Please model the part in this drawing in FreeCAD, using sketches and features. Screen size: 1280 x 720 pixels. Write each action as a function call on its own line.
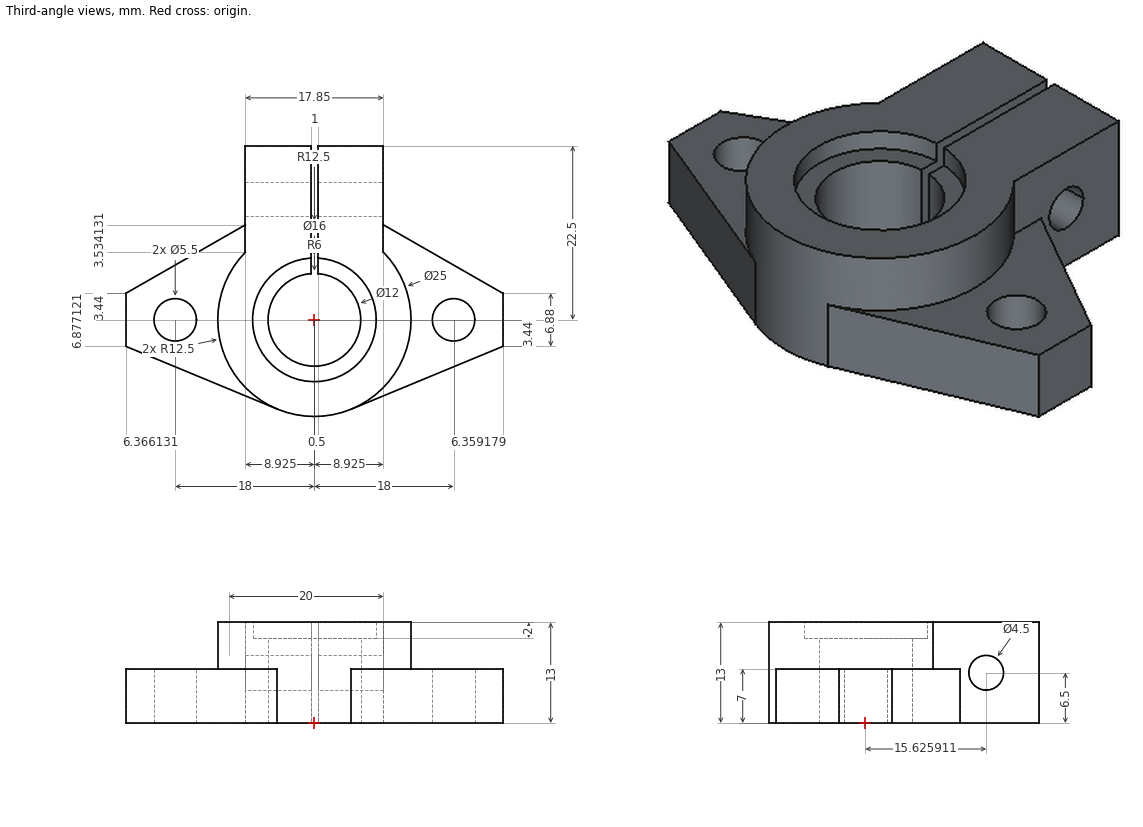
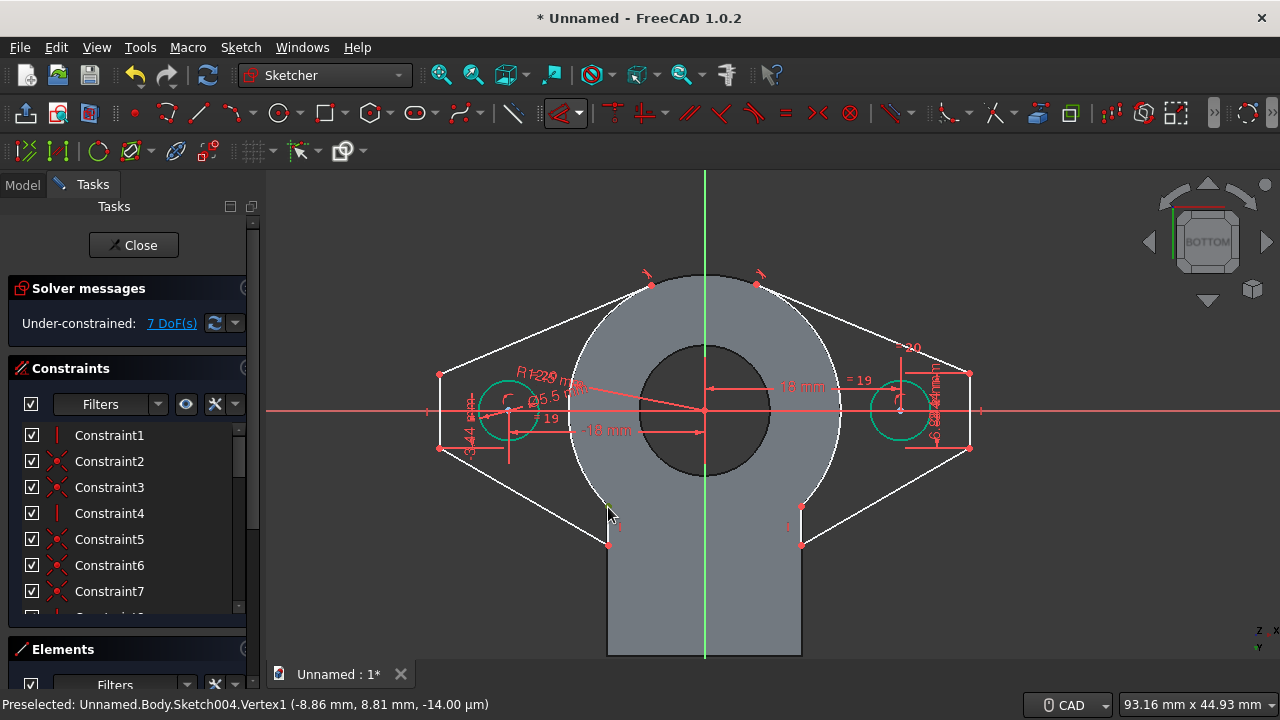
click(582, 114)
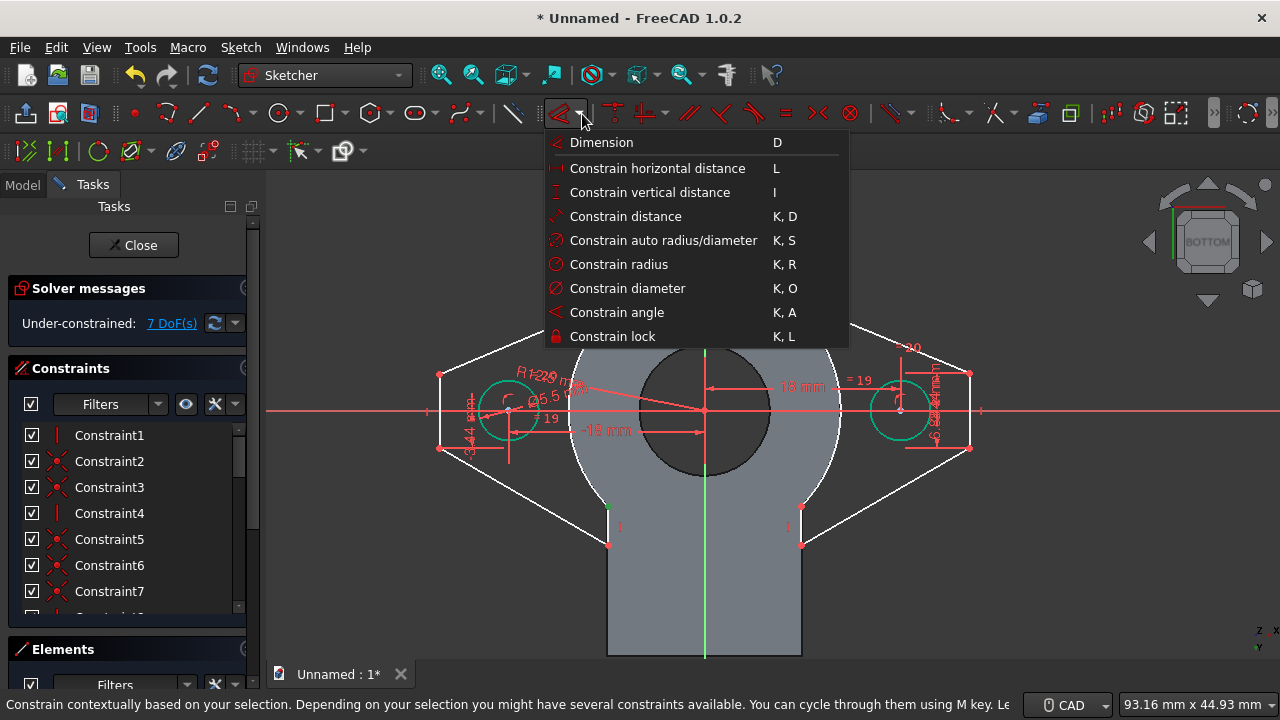
click(697, 168)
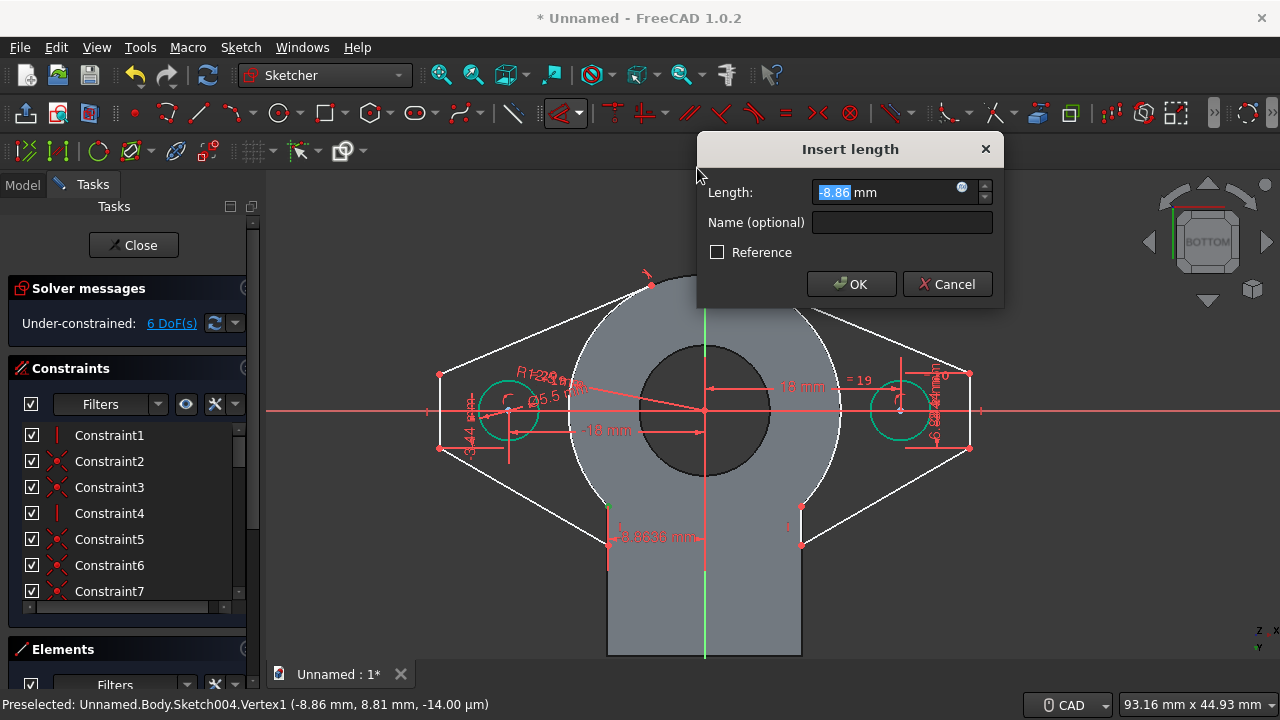
text(-8.925)
key(Return)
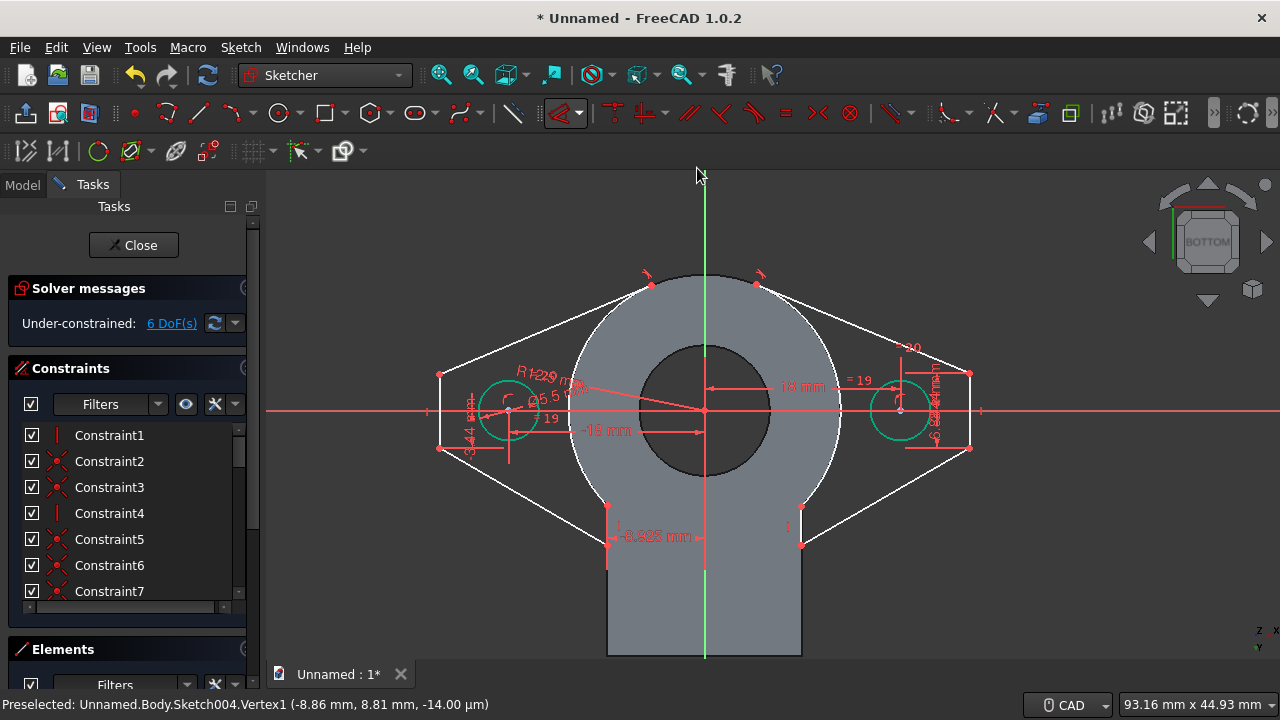
click(801, 546)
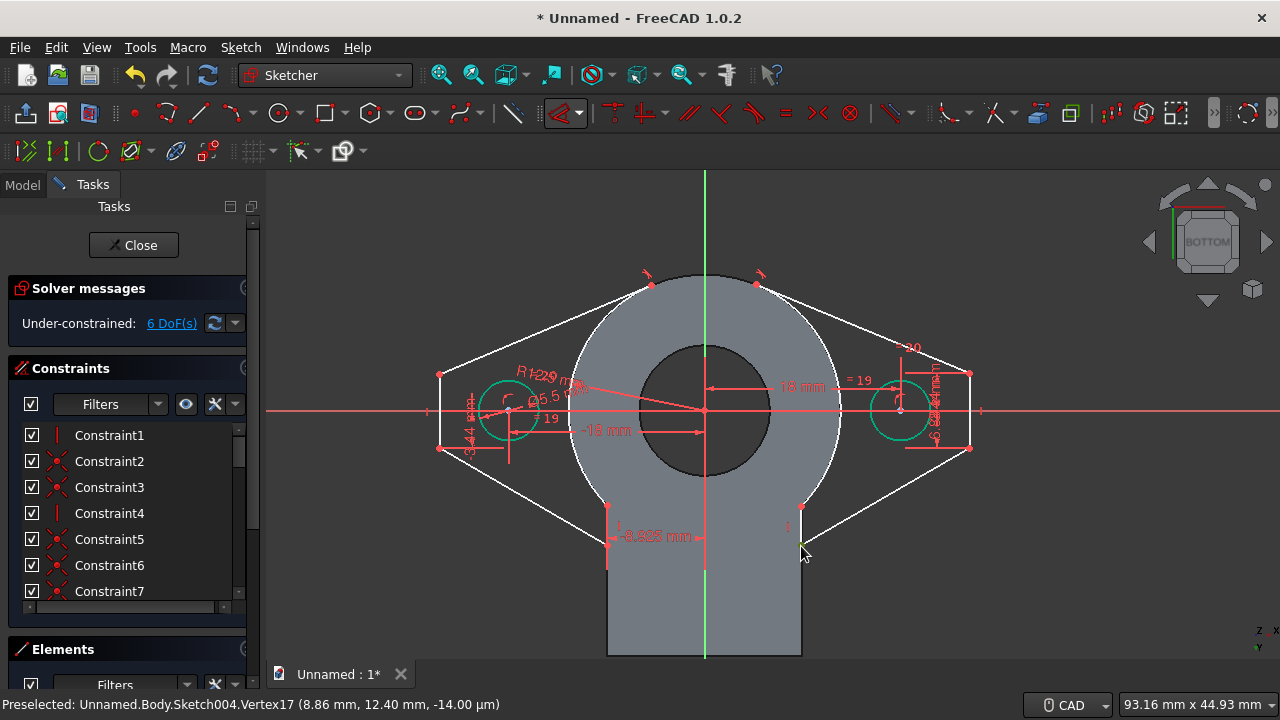
key(l)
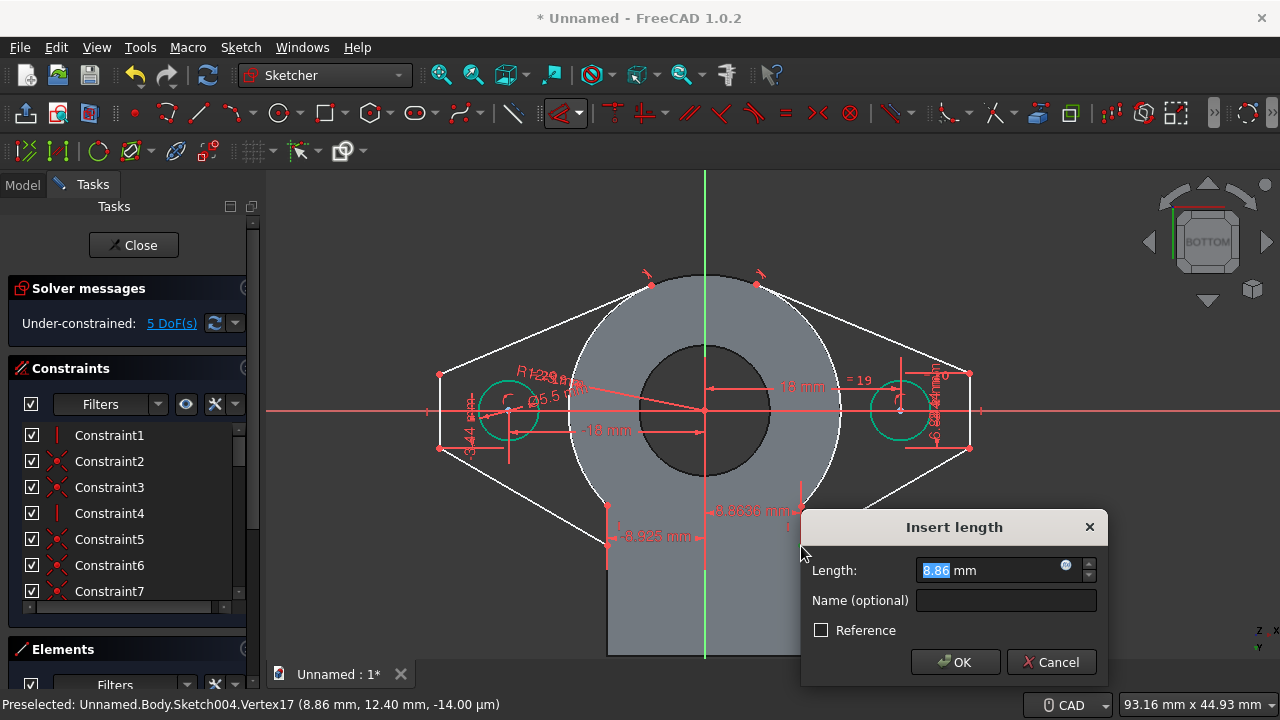
text(8.925)
key(Return)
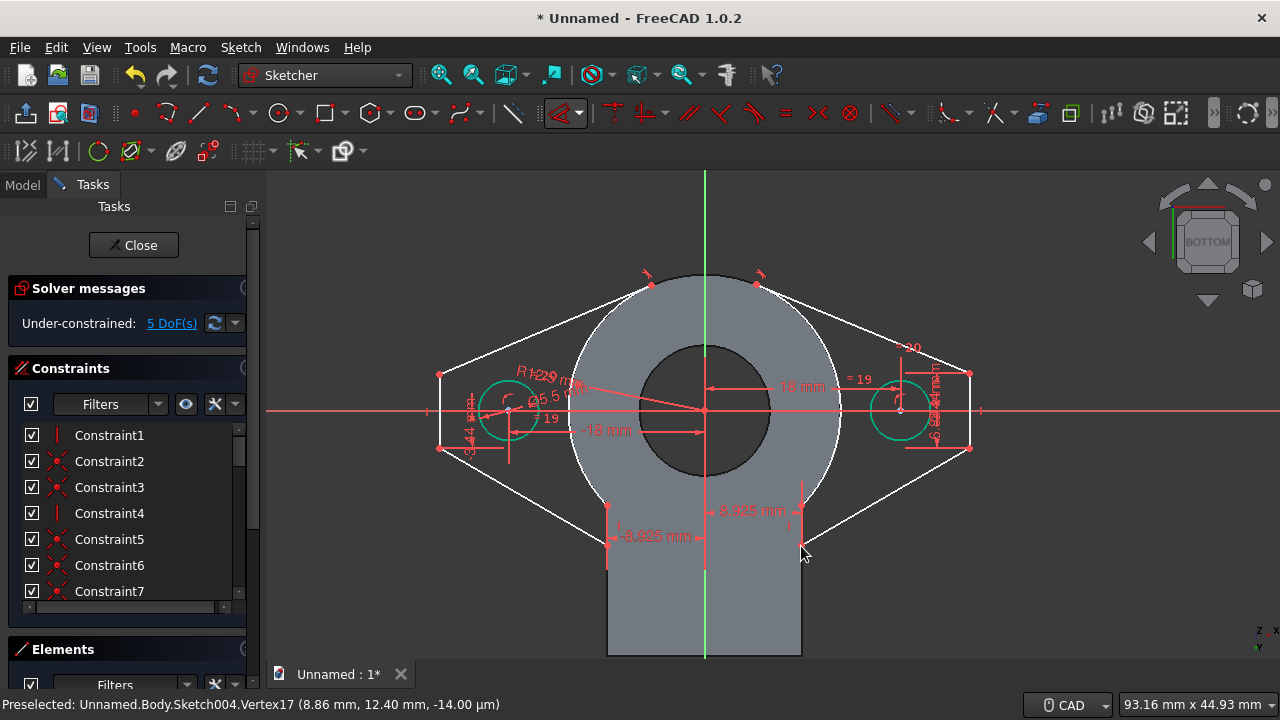
click(607, 518)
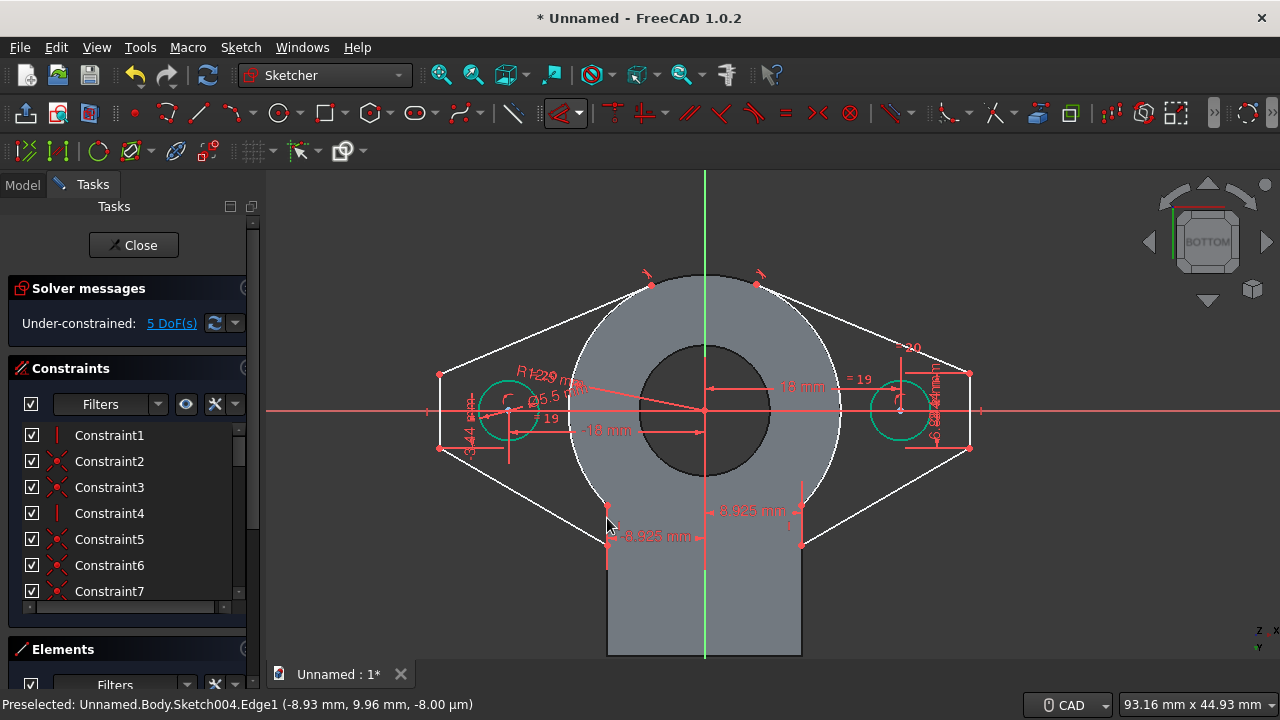
key(i)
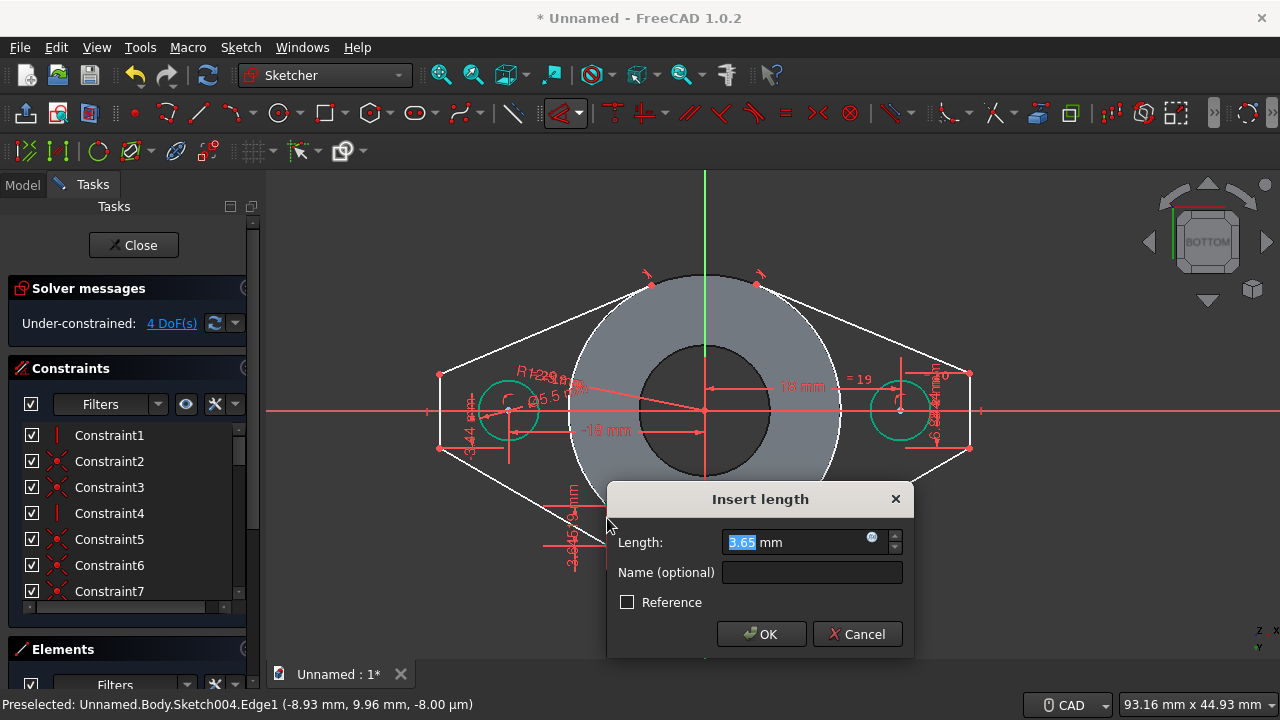
text(3.534131)
key(Return)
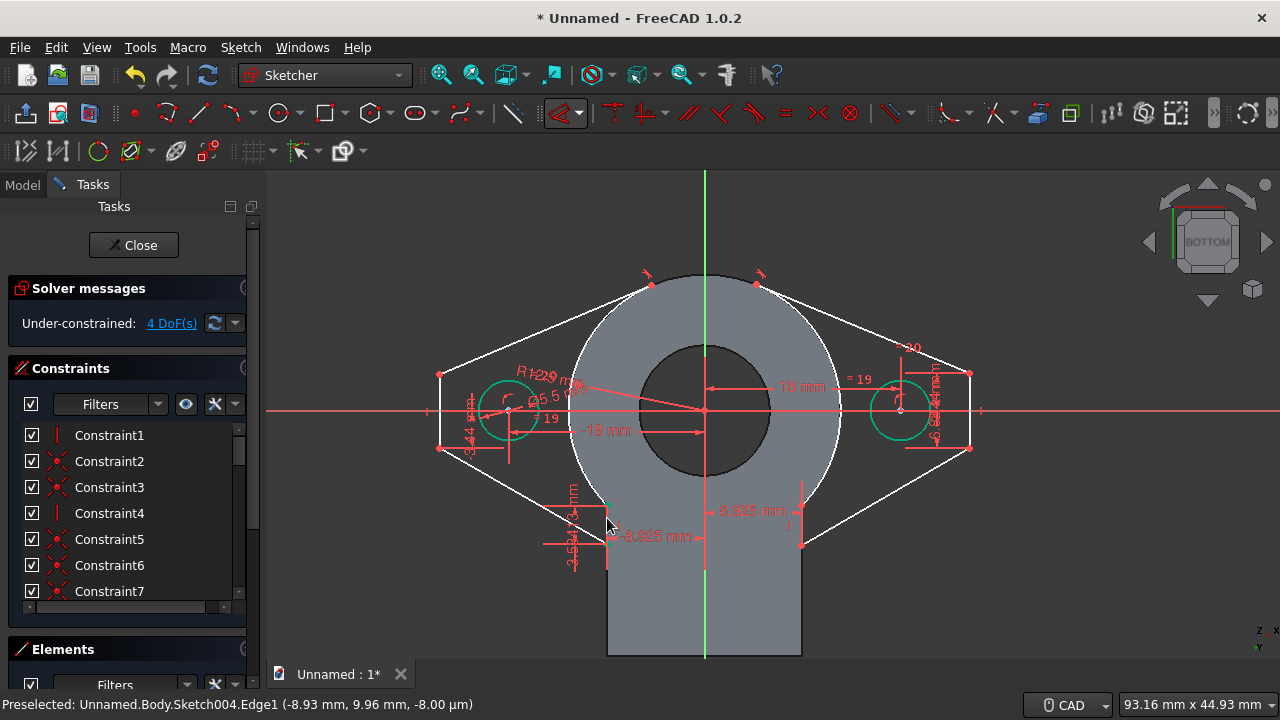
click(440, 426)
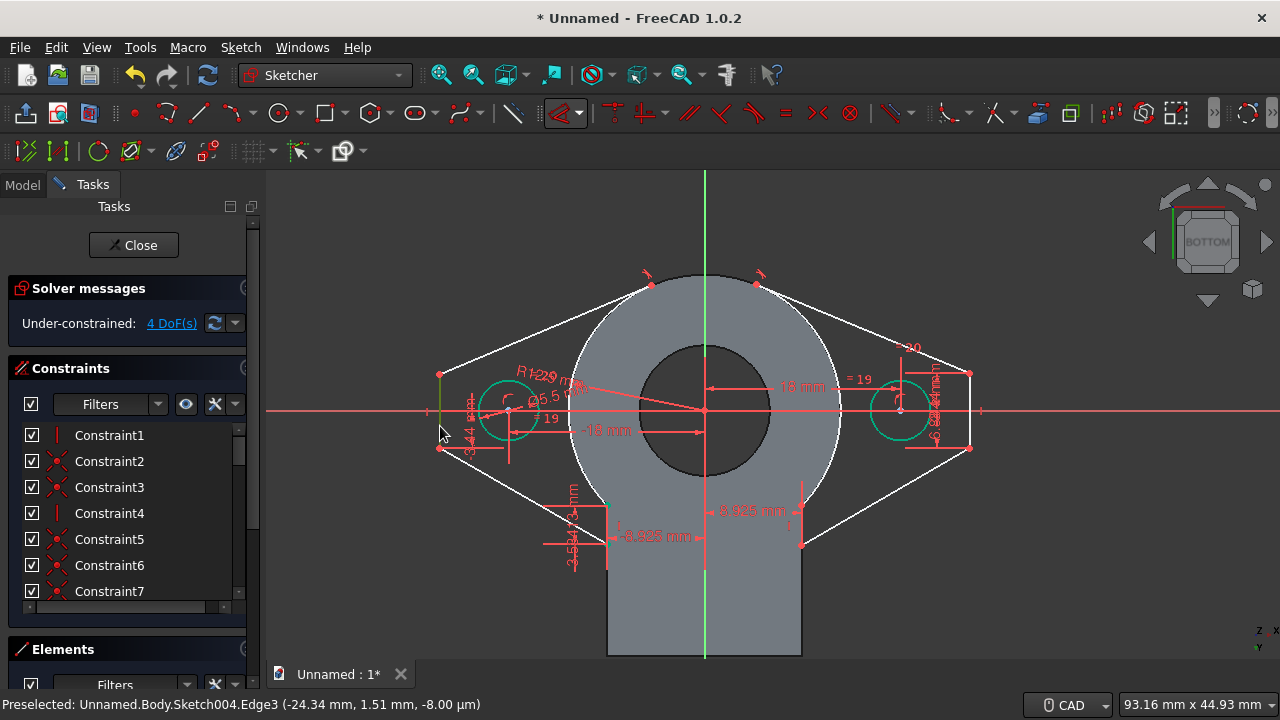
click(582, 114)